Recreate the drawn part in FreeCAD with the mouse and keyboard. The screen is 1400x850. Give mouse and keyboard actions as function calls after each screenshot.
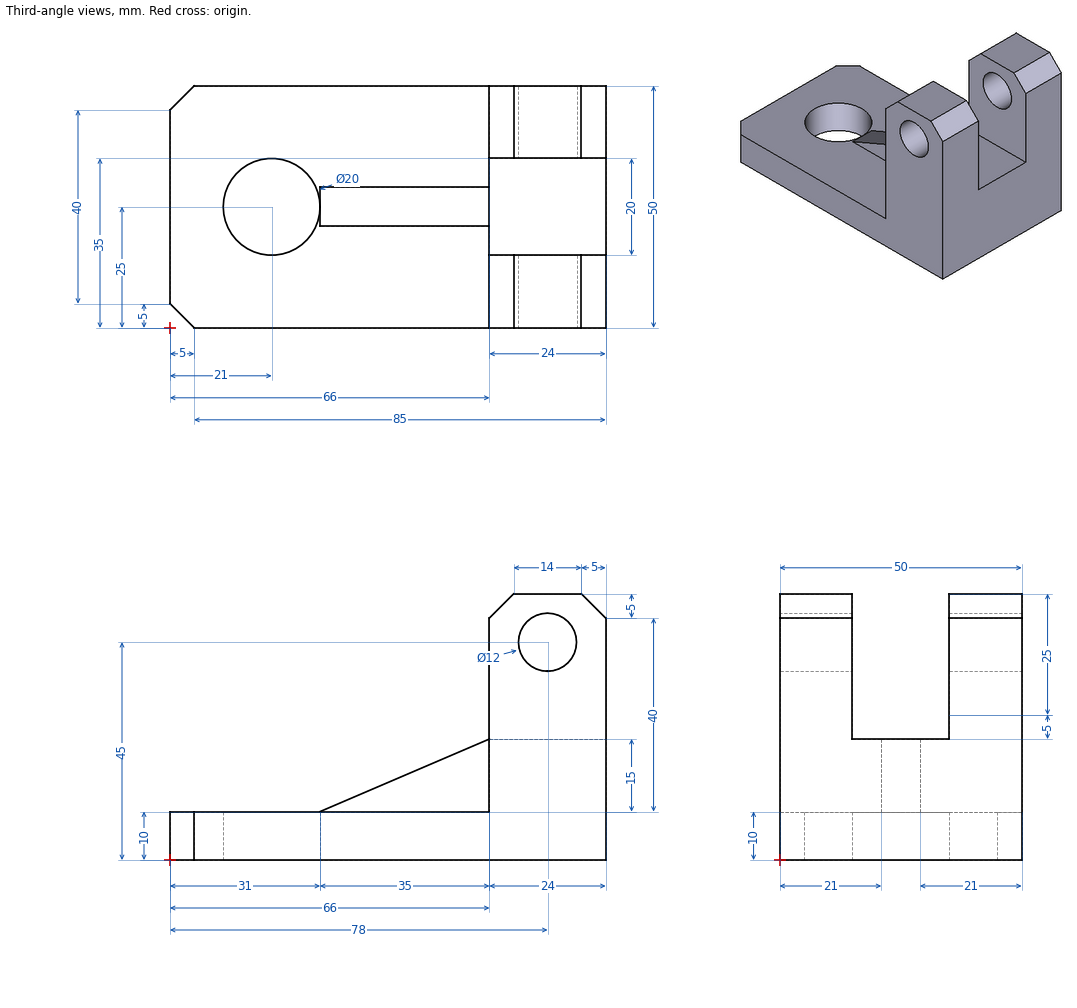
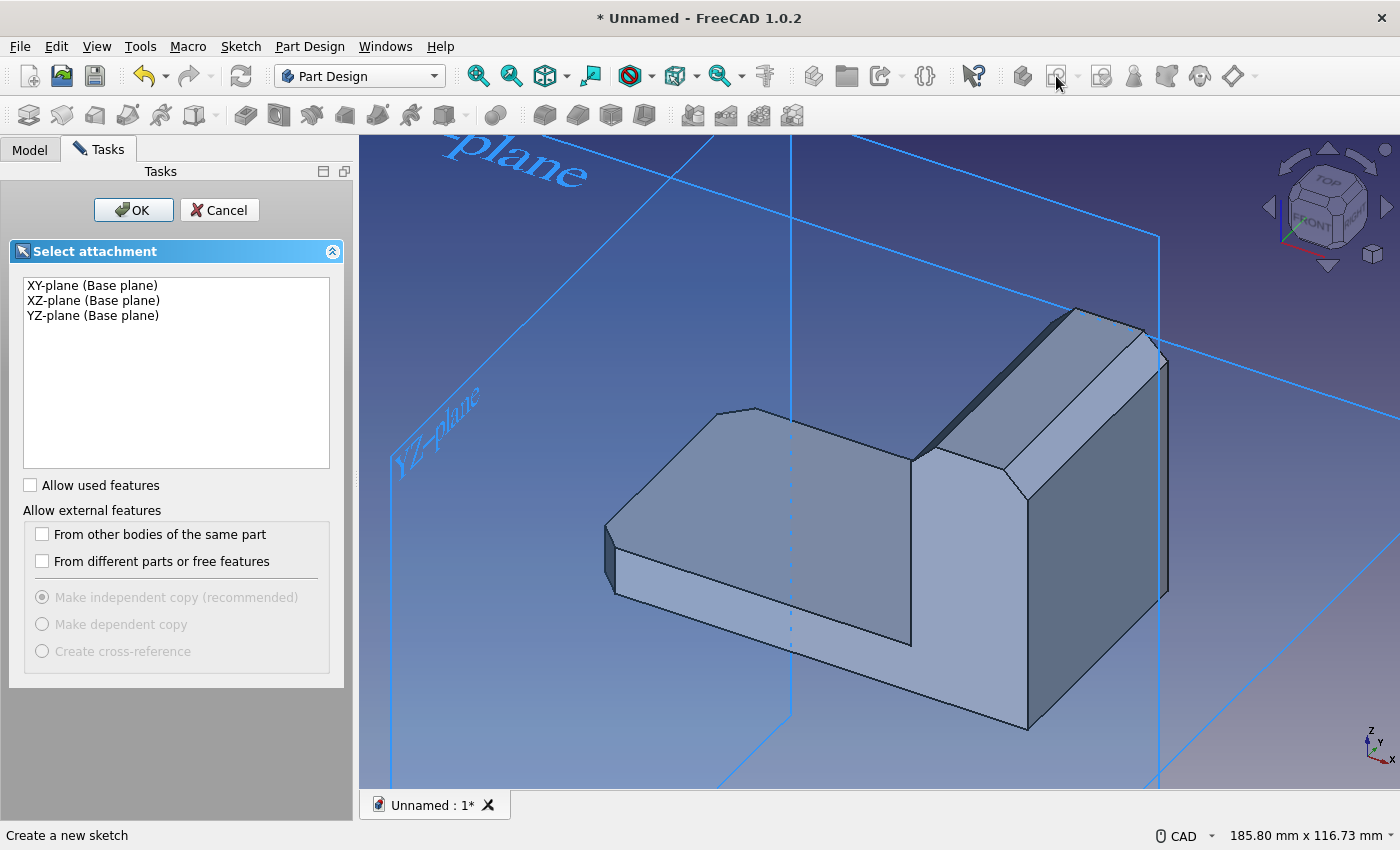
click(84, 300)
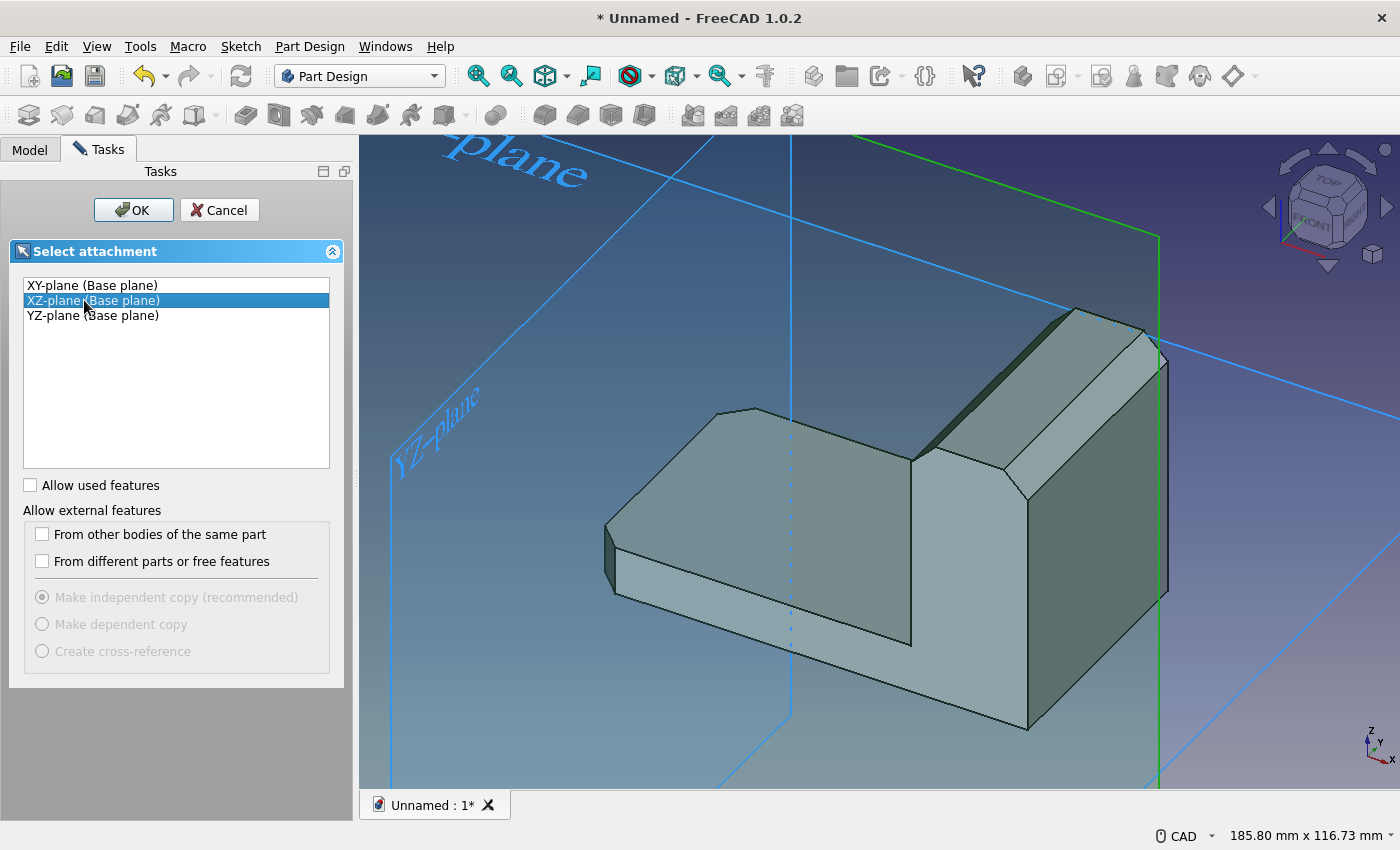
click(134, 210)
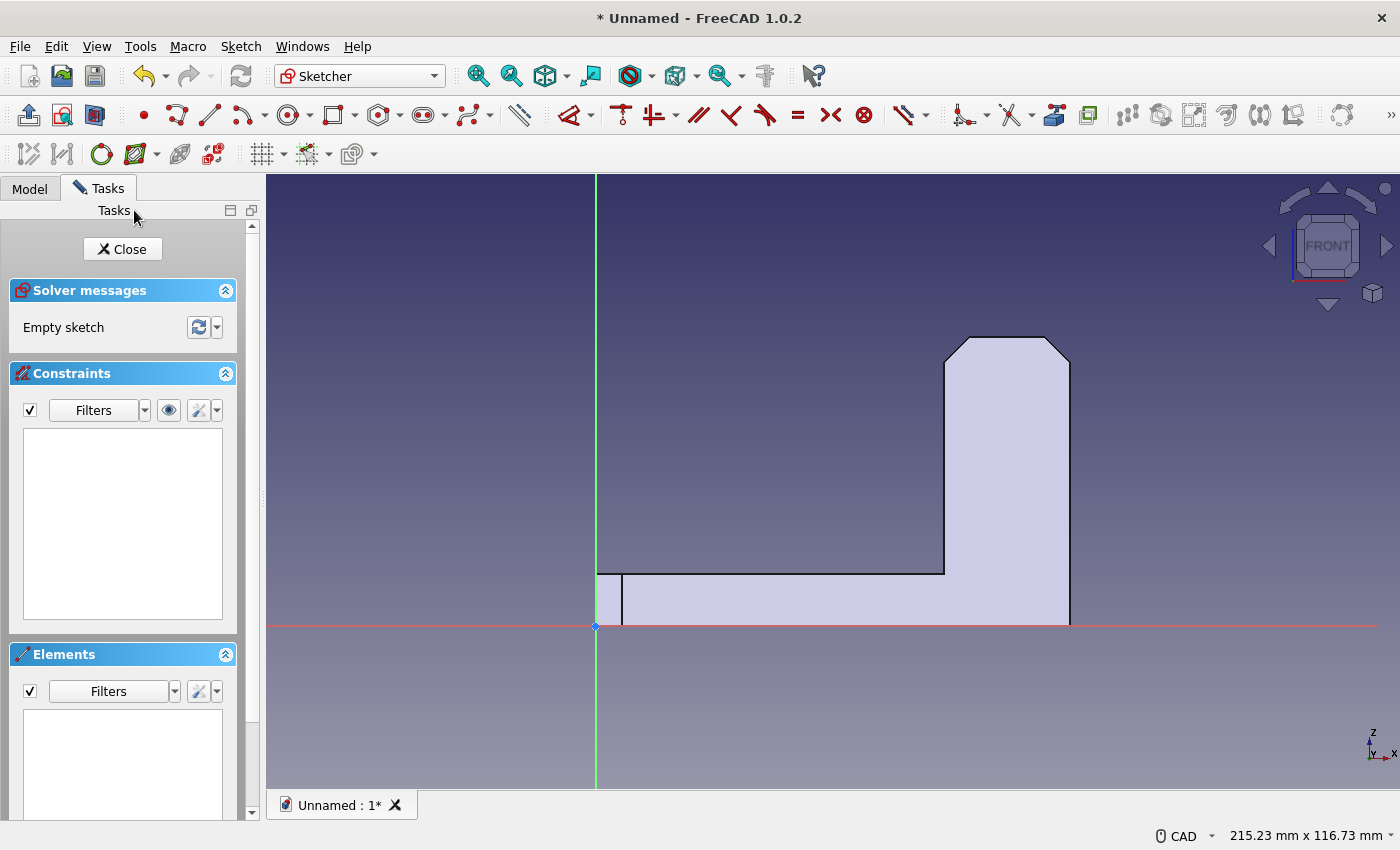
scroll(1055, 371, up, 9)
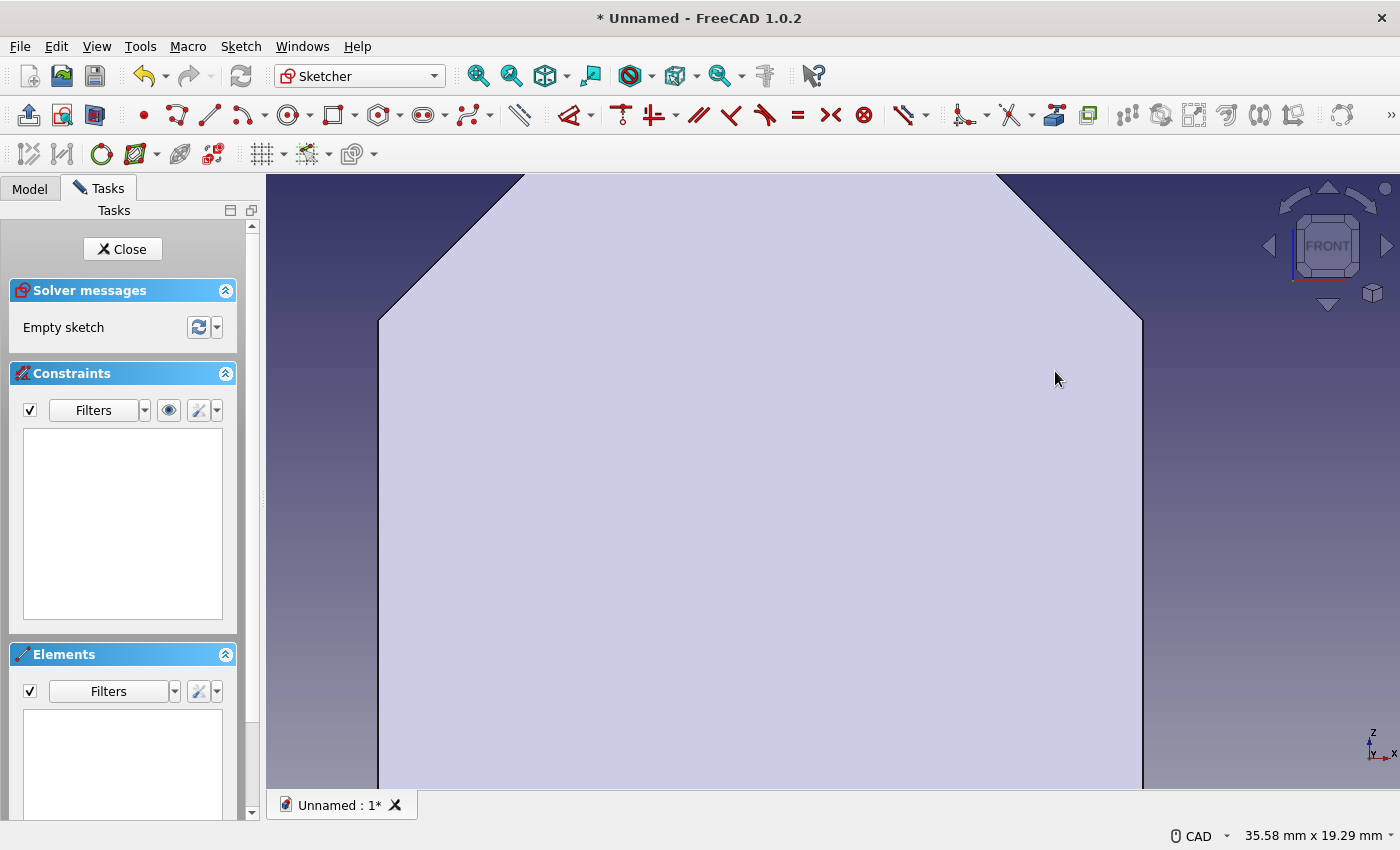
click(288, 116)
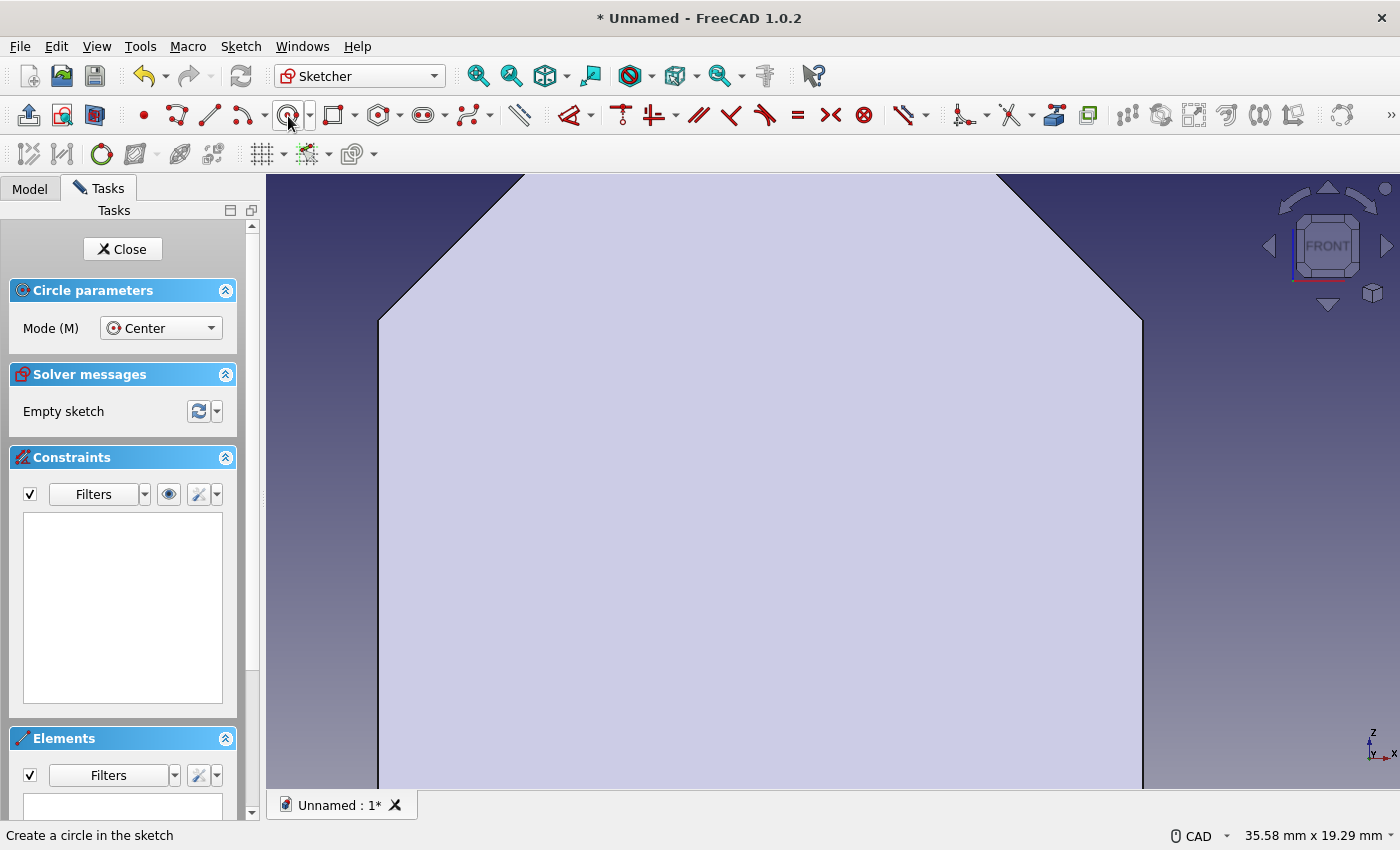
click(760, 480)
move(896, 345)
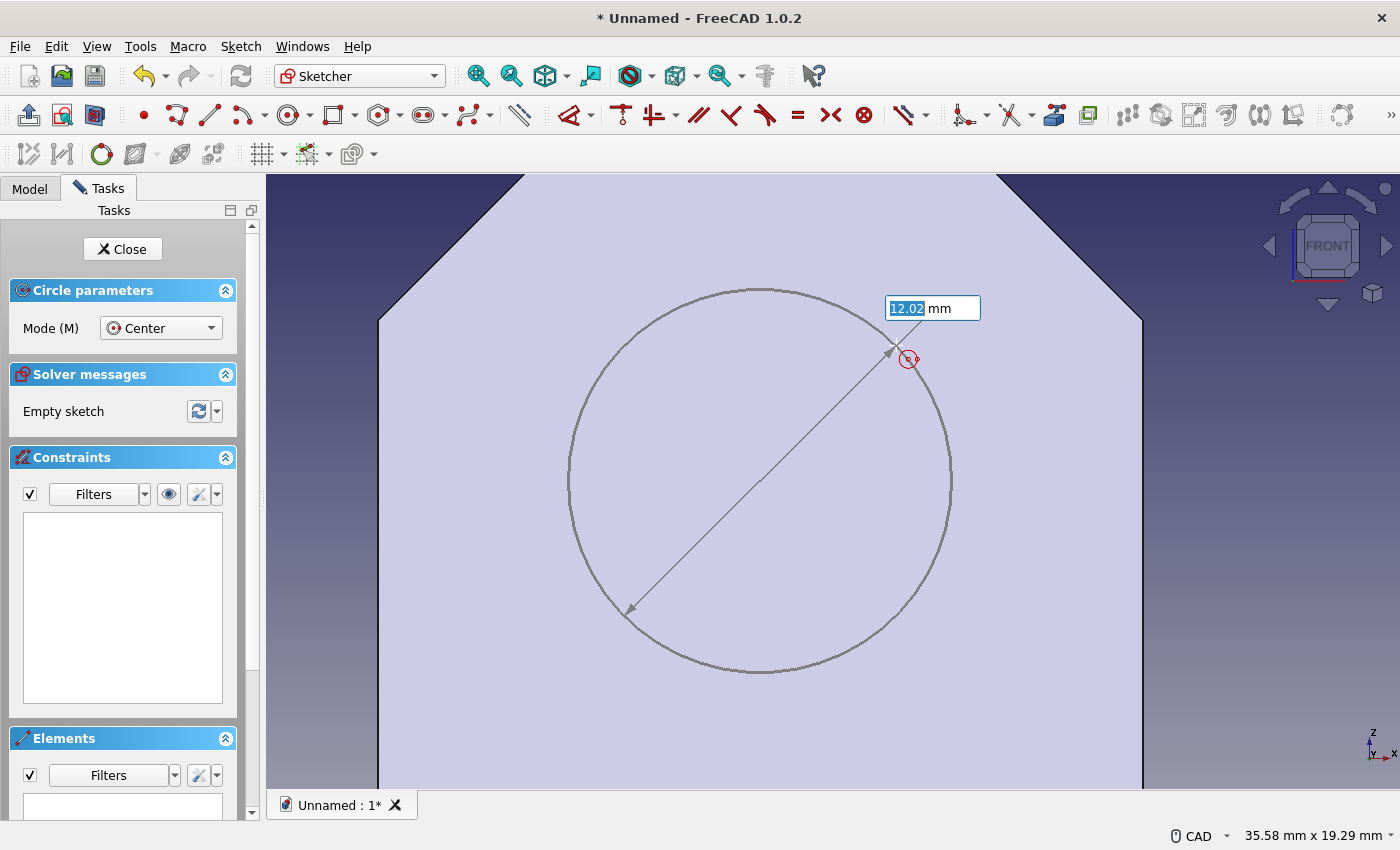
text(12)
key(Return)
key(Escape)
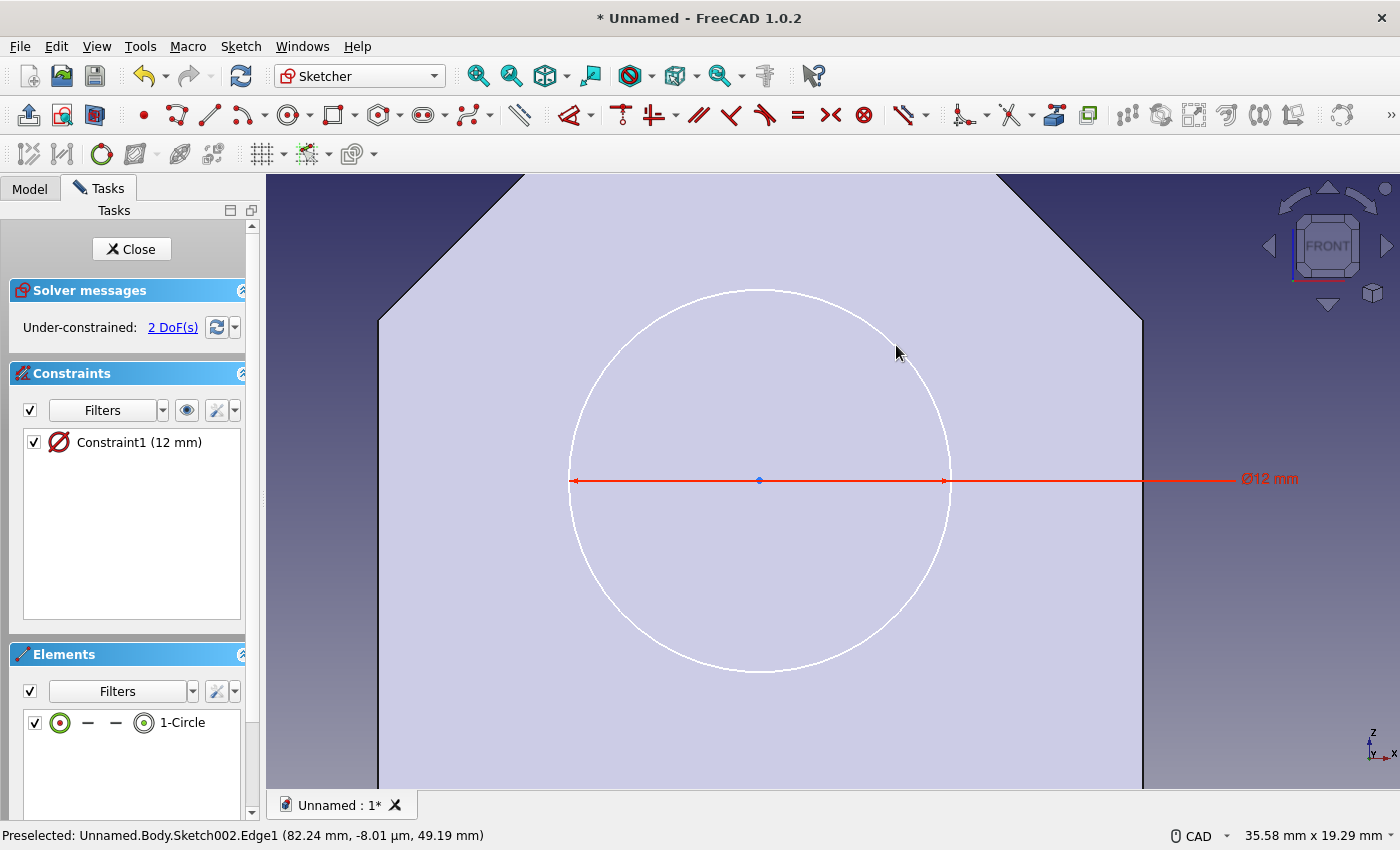
click(568, 116)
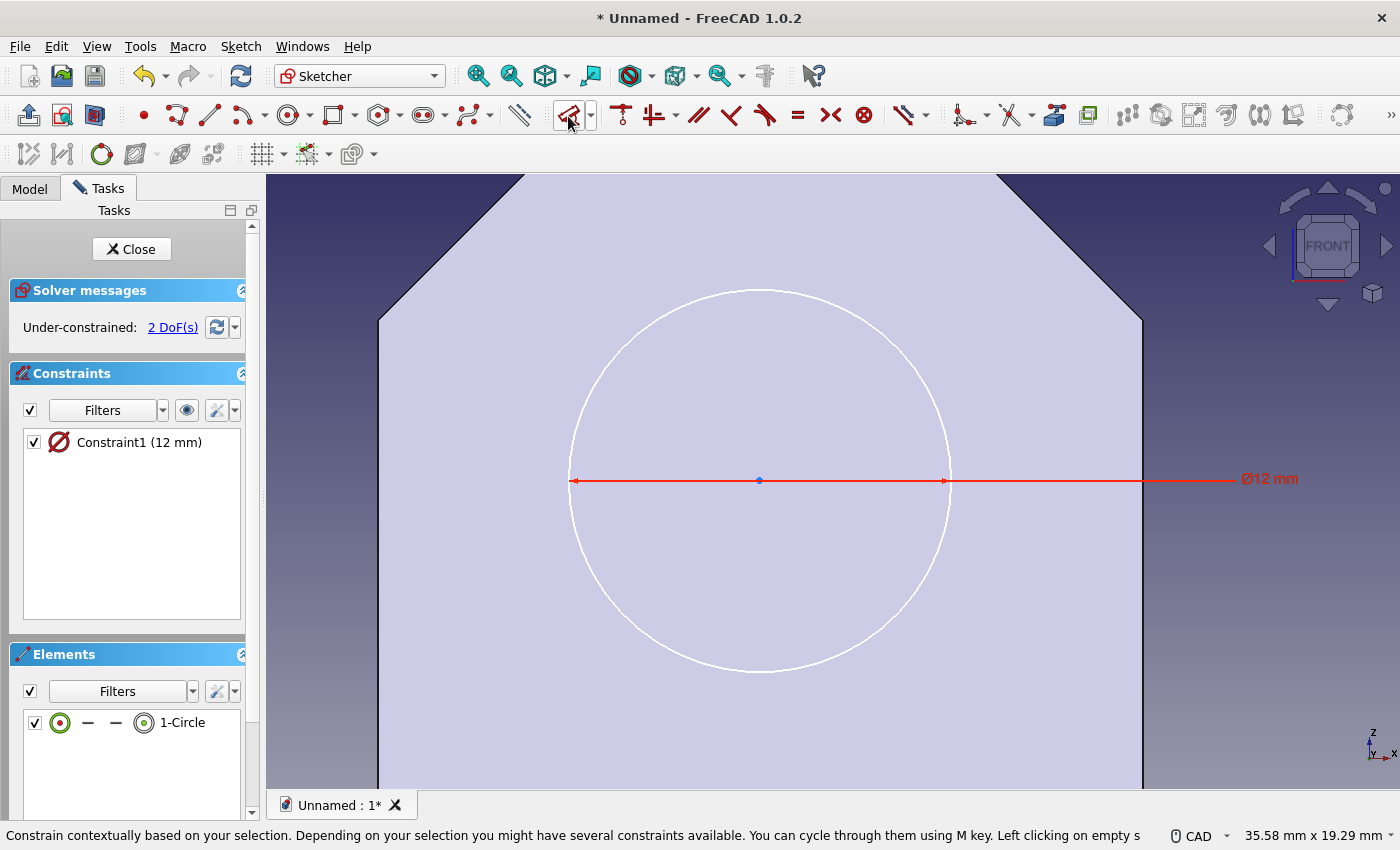
click(760, 481)
click(527, 447)